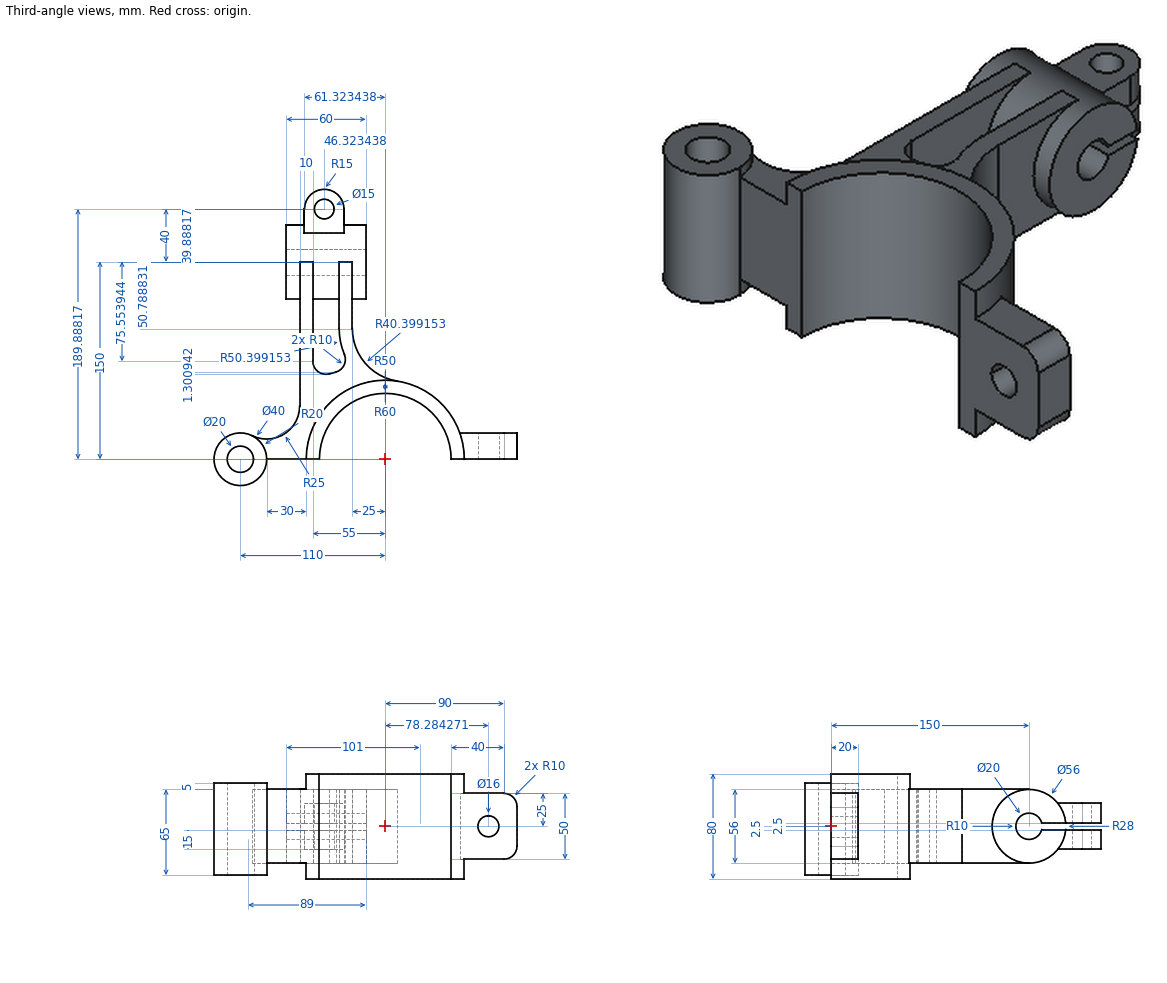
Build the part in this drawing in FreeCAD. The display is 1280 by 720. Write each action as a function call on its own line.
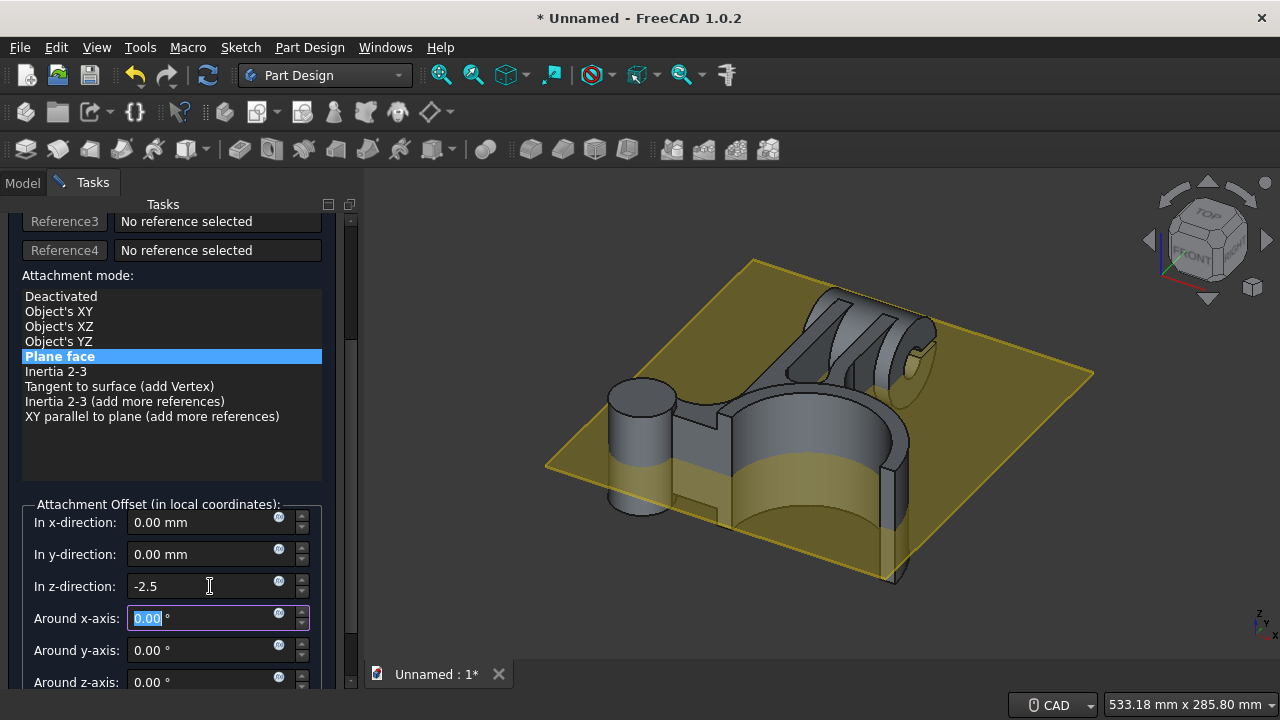
scroll(351, 451, up, 4)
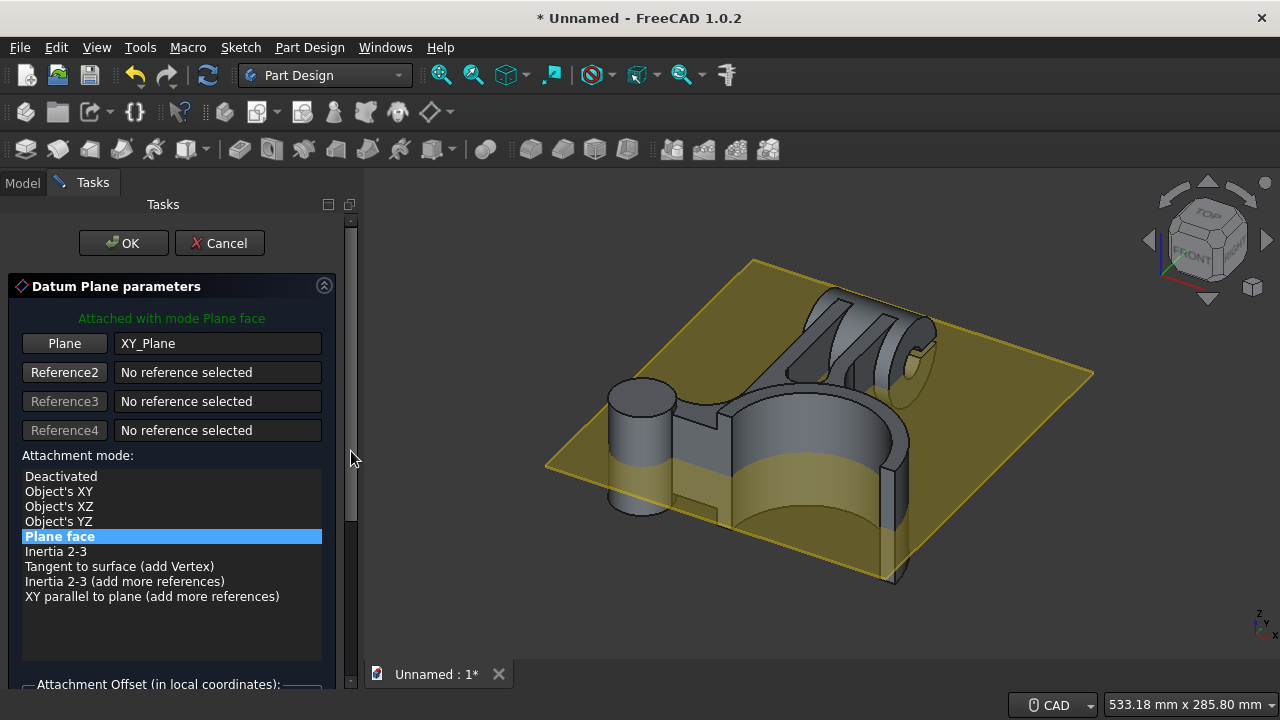
click(124, 243)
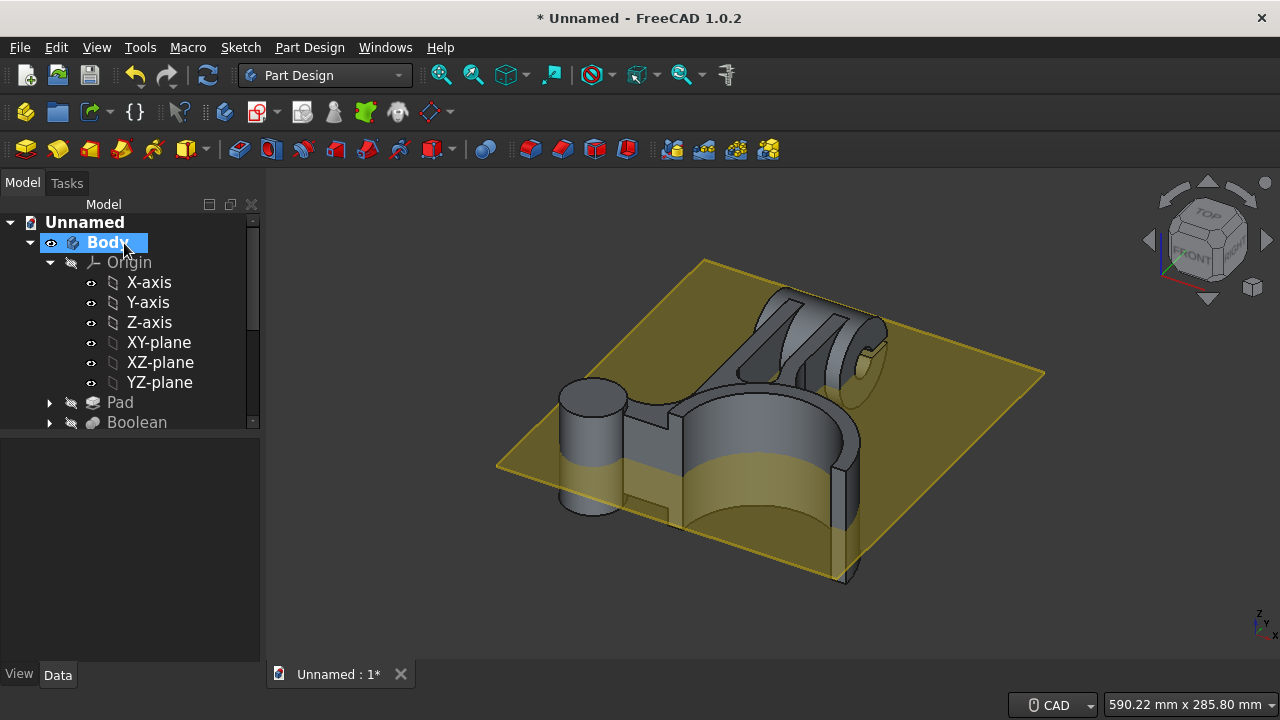
scroll(100, 318, down, 3)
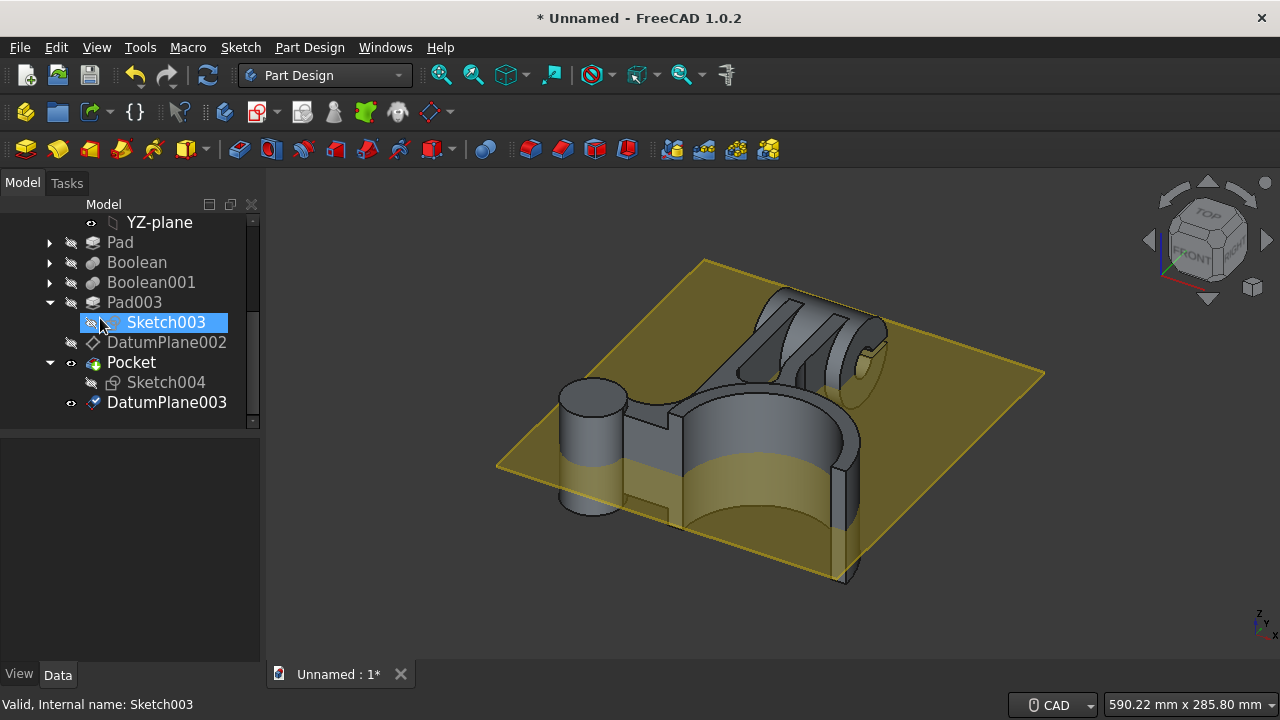
click(116, 403)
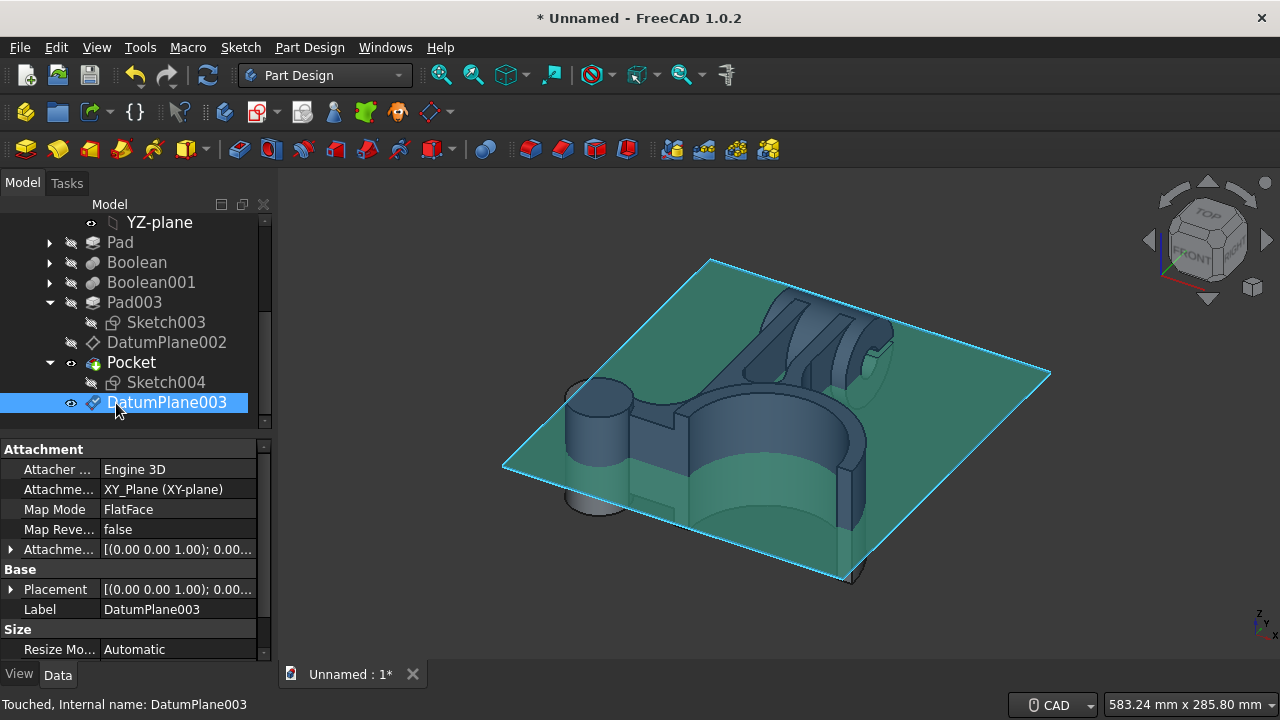
click(258, 112)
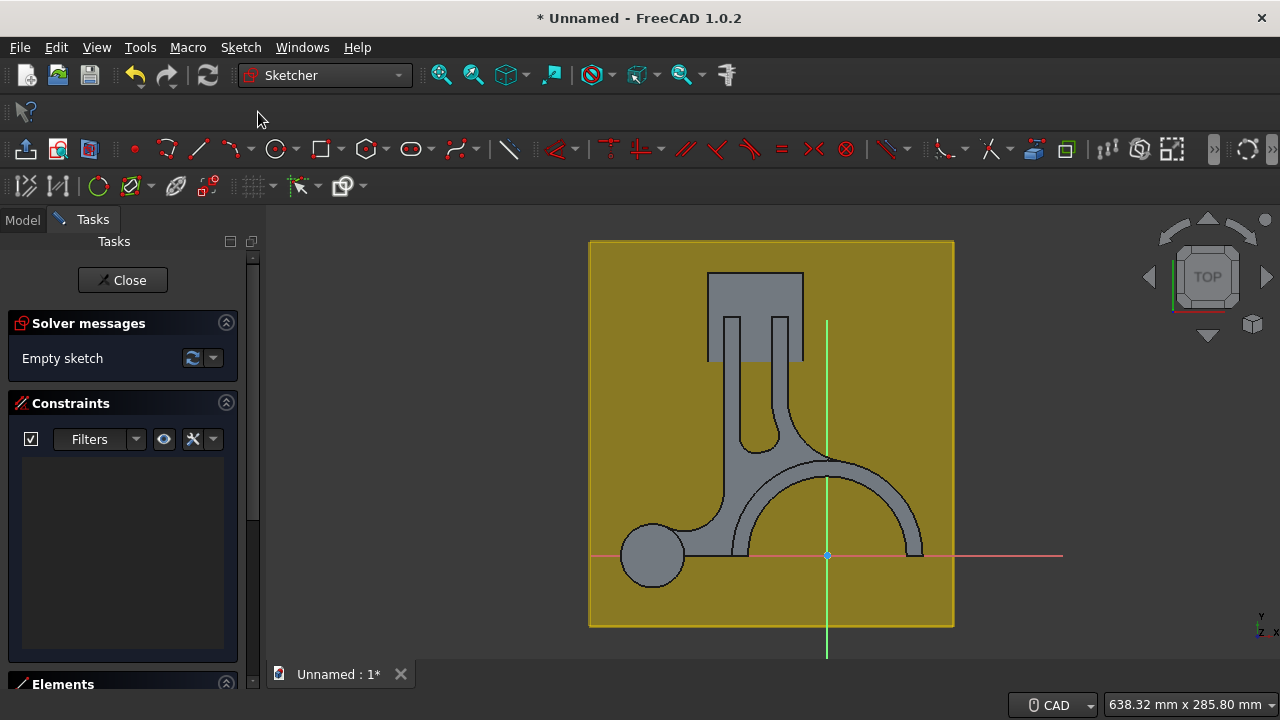
key(q)
key(s)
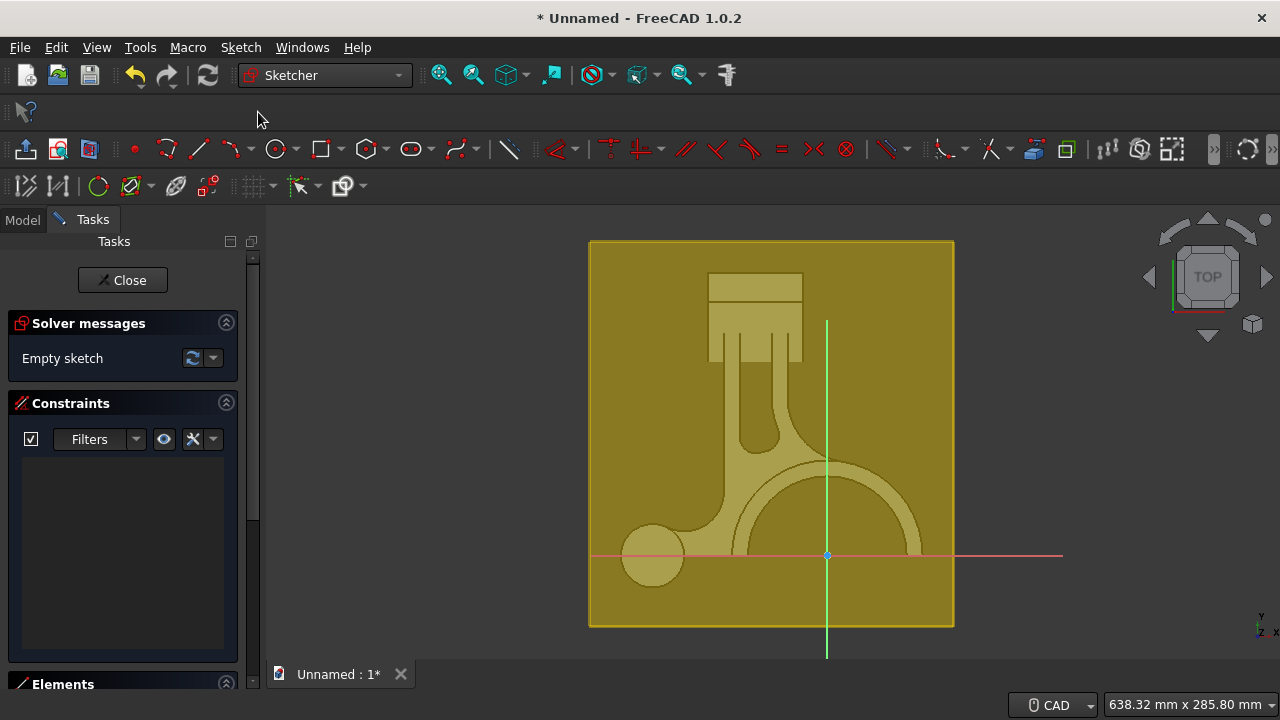
scroll(704, 432, down, 5)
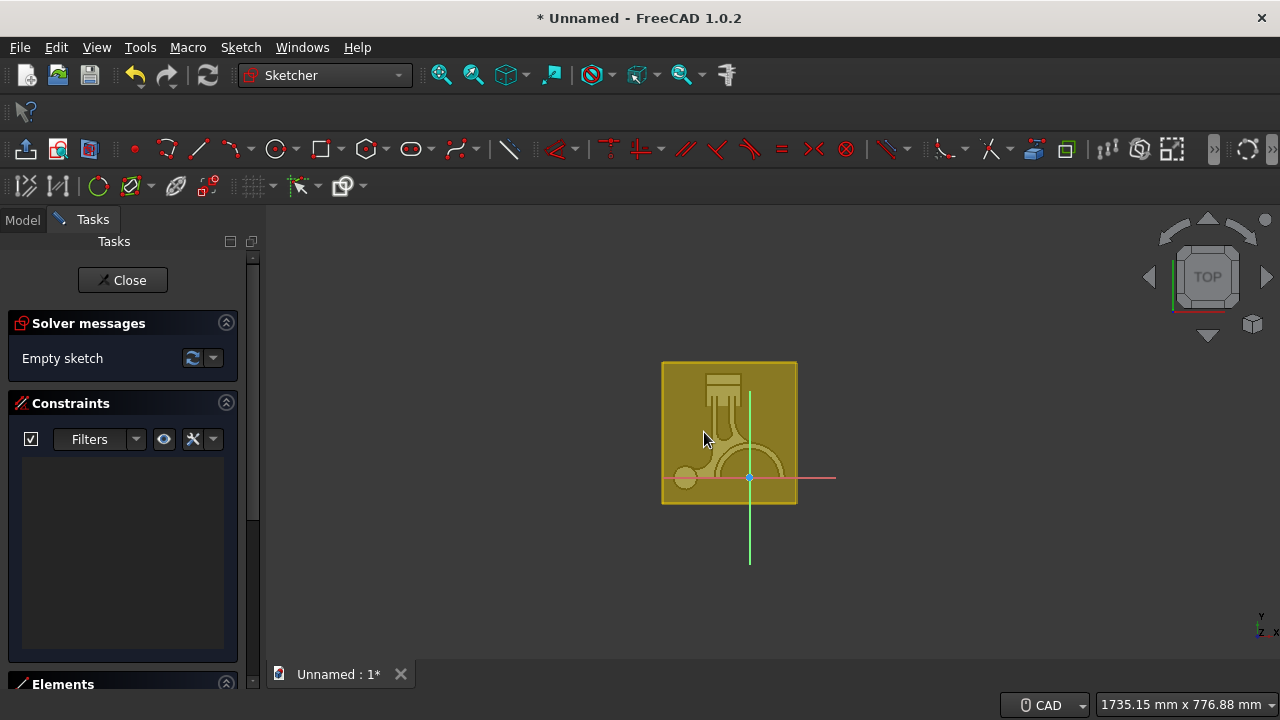
scroll(725, 367, up, 11)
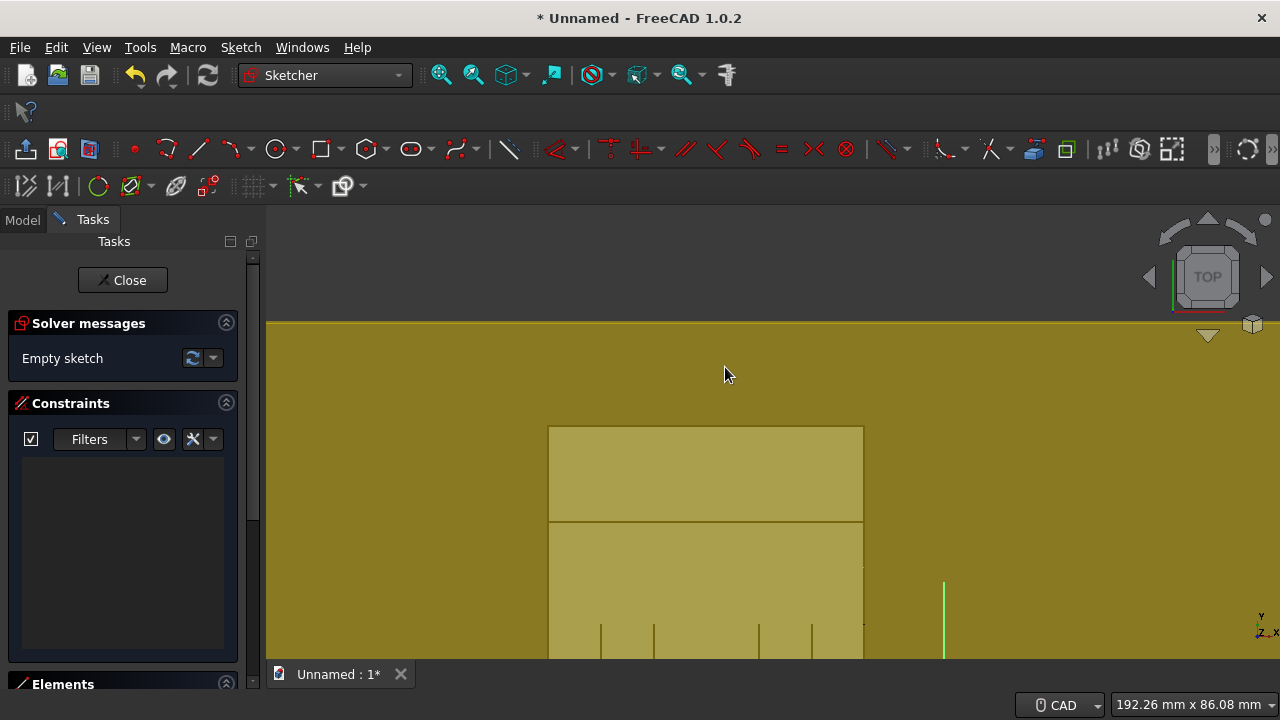
key(g)
key(m)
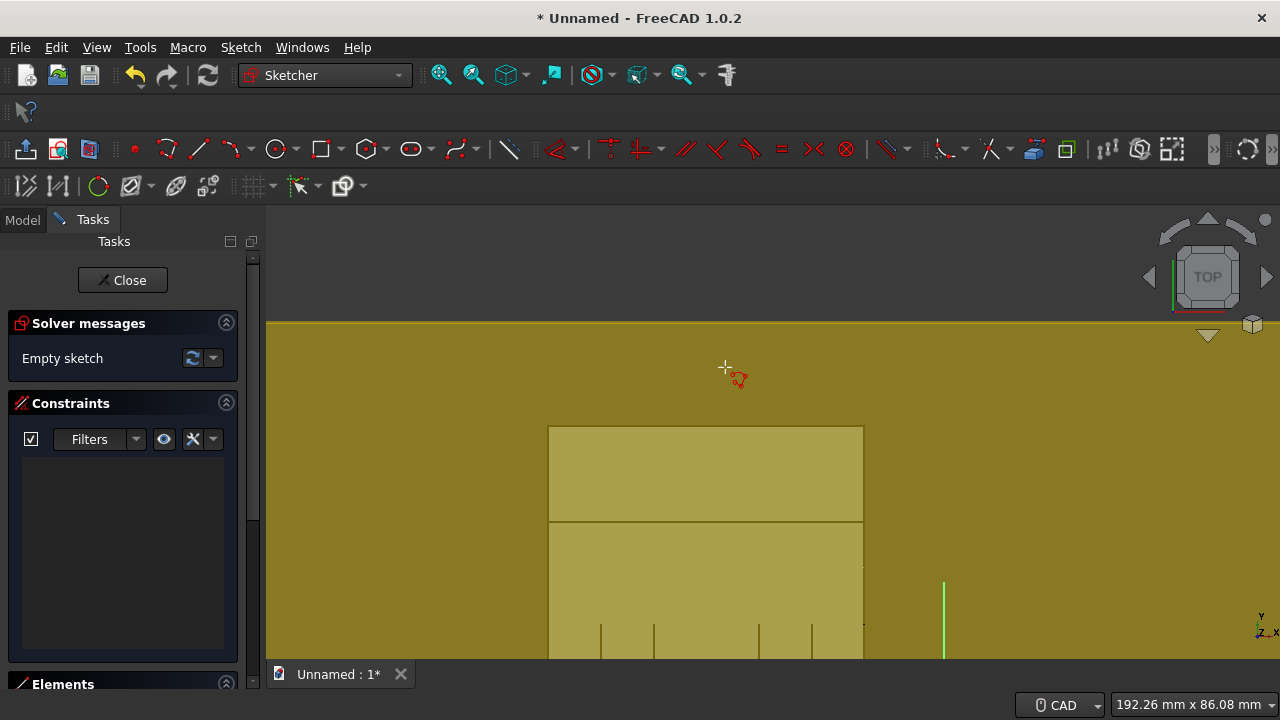
click(620, 363)
click(620, 573)
click(778, 582)
click(778, 363)
right_click(778, 363)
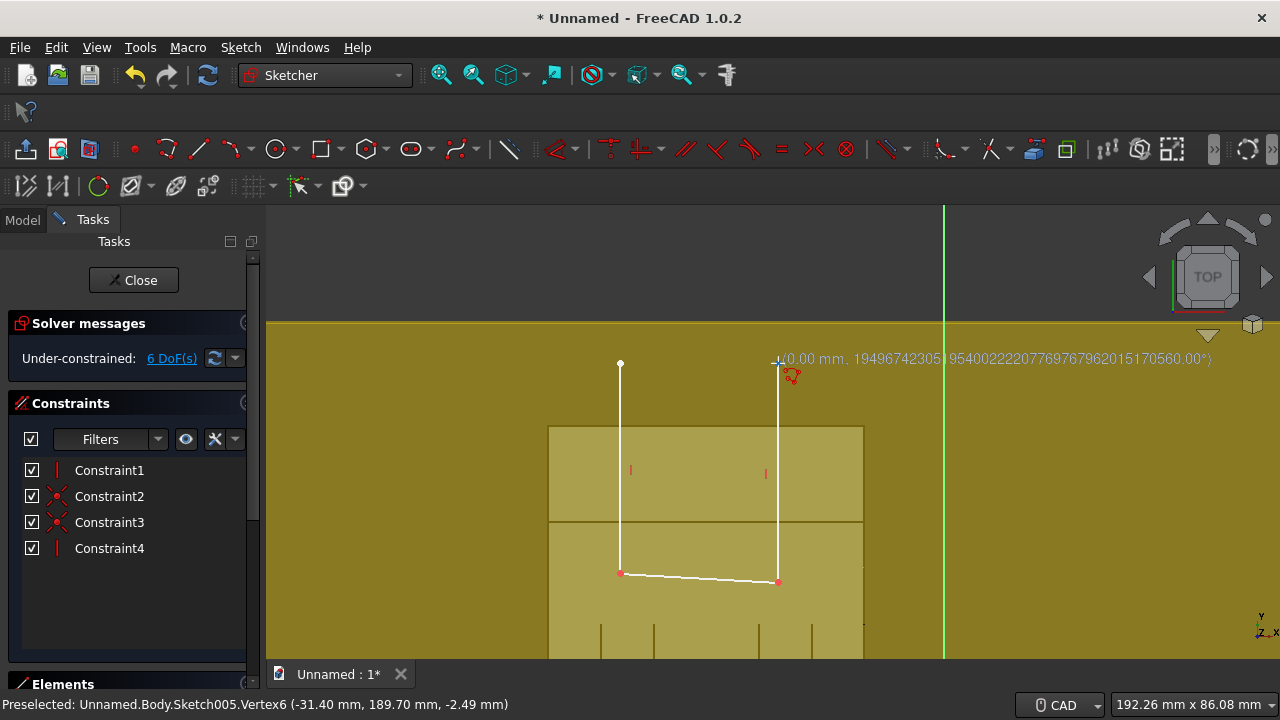
key(g)
key(3)
key(a)